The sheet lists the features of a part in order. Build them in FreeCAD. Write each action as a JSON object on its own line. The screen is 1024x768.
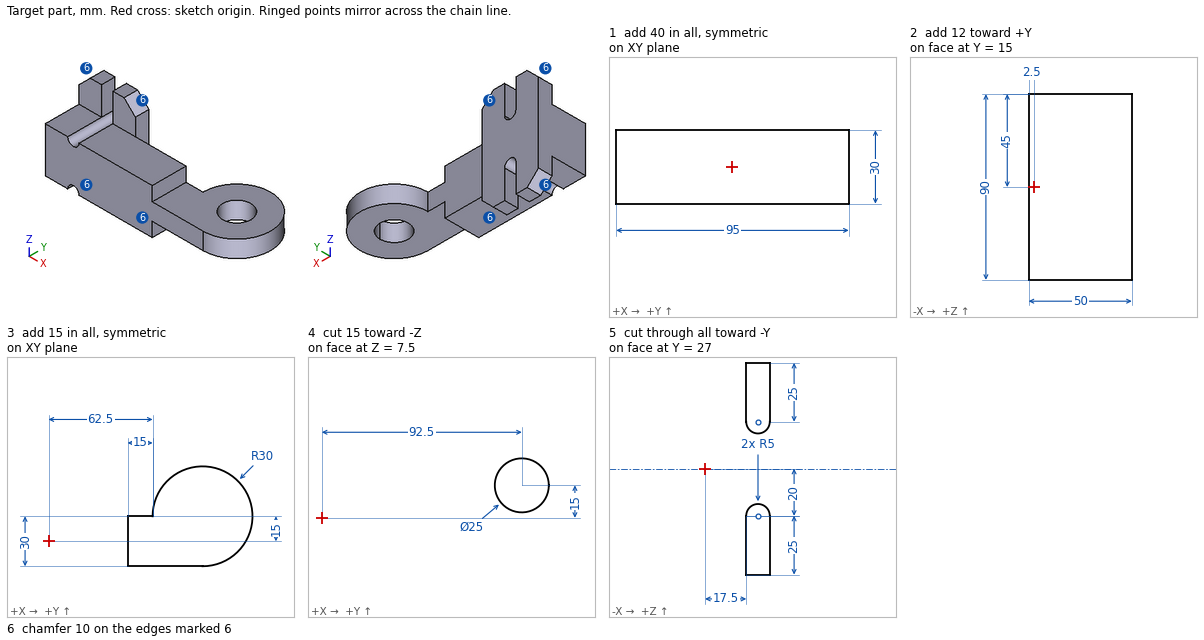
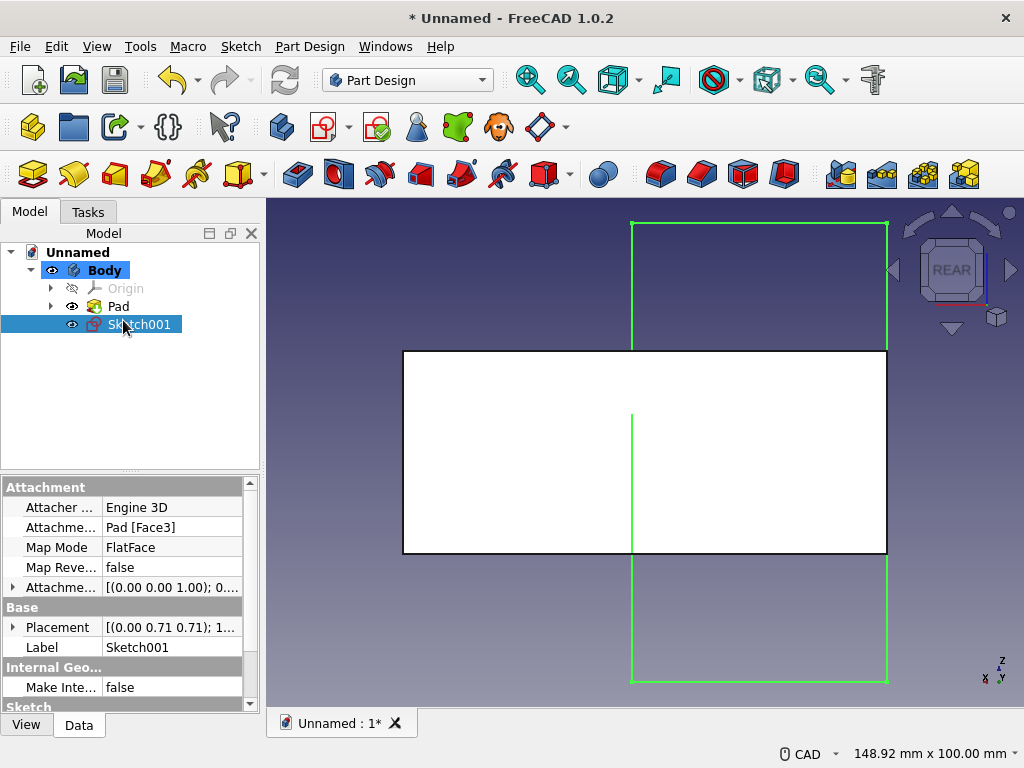
{"action": "left_click", "coordinate": [33, 174]}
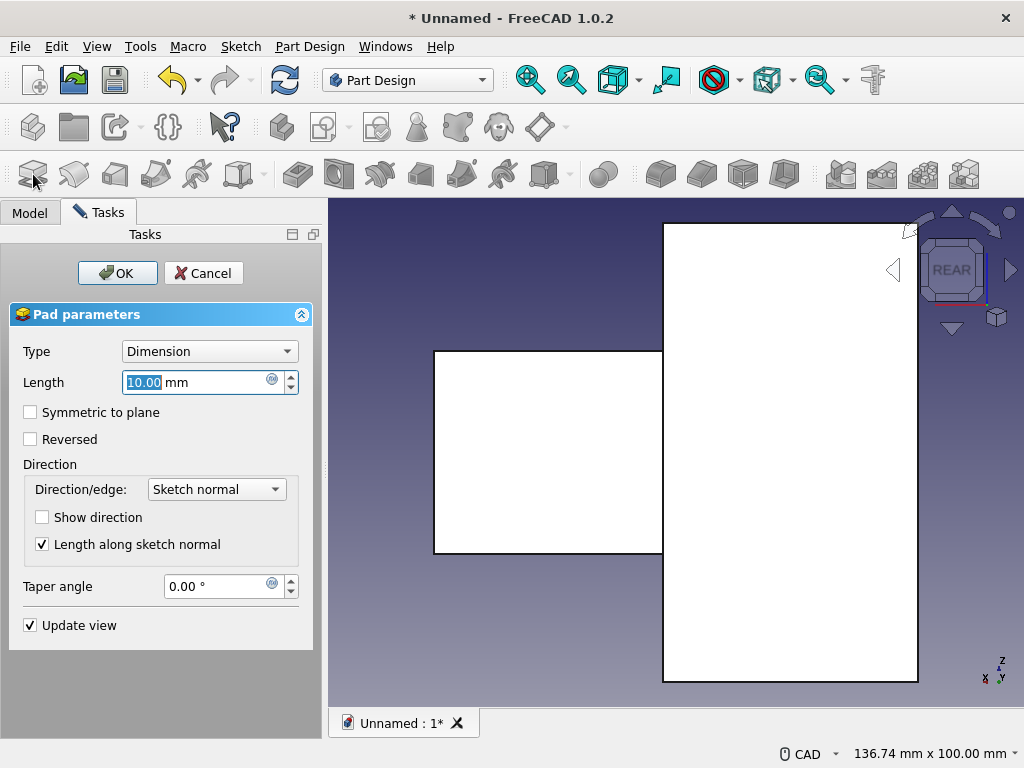
{"action": "type", "text": "12"}
{"action": "key", "text": "Tab"}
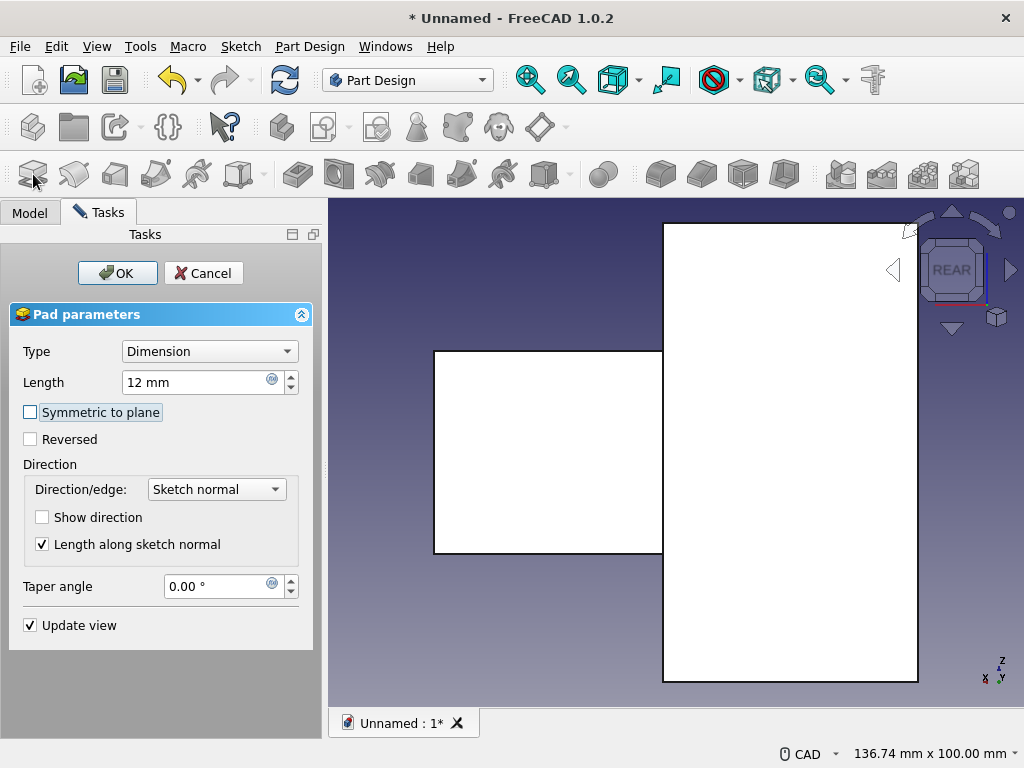
{"action": "left_click", "coordinate": [118, 273]}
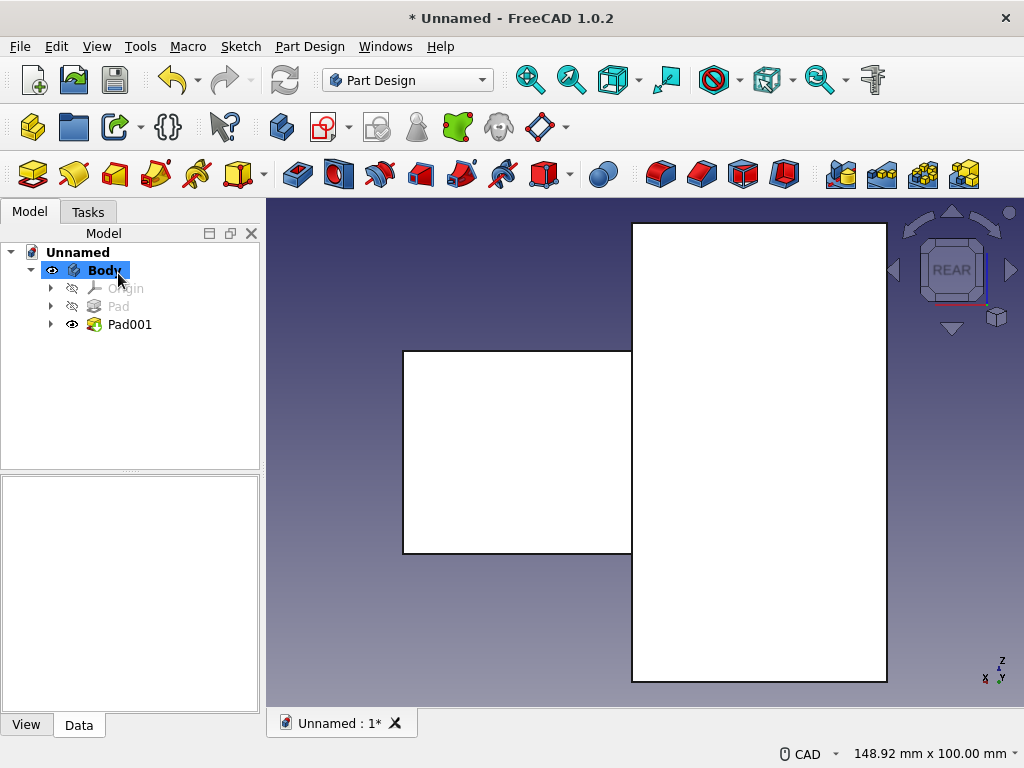
{"action": "left_click", "coordinate": [322, 128]}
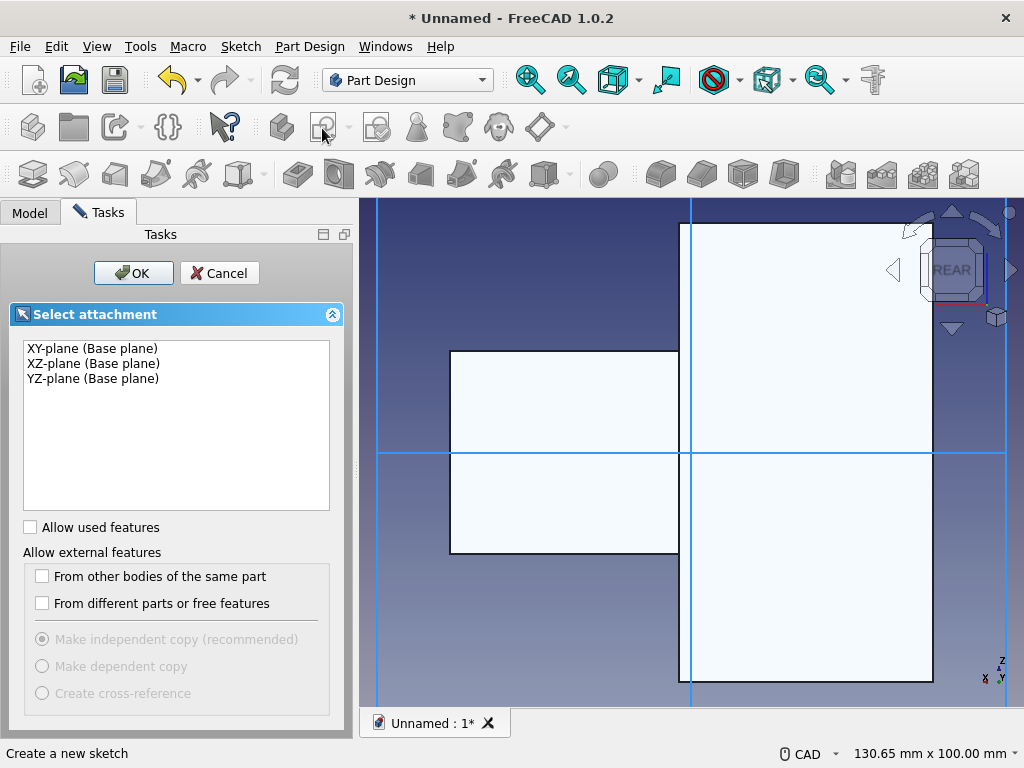
{"action": "left_click", "coordinate": [84, 348]}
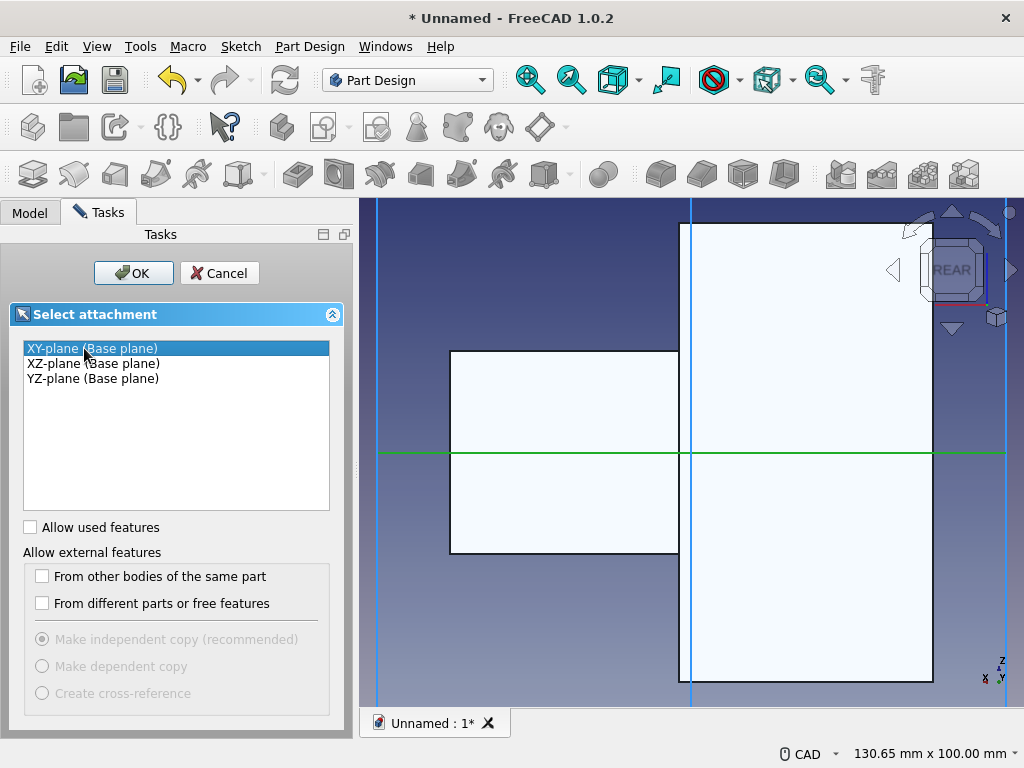
{"action": "left_click", "coordinate": [134, 273]}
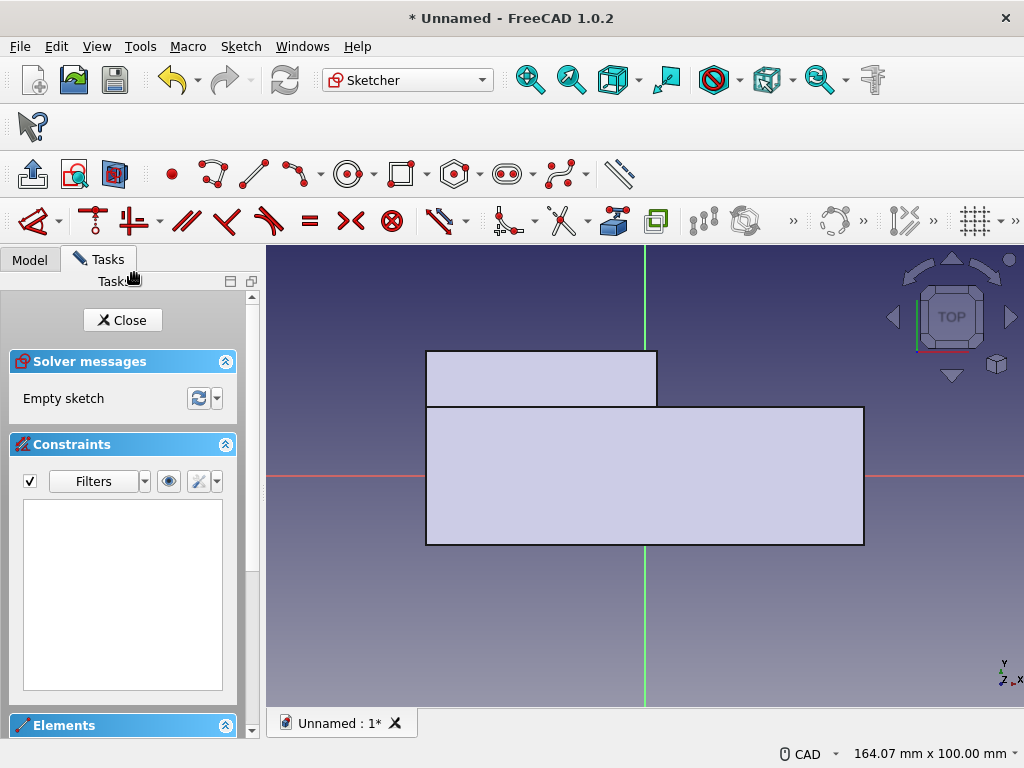
{"action": "left_click", "coordinate": [115, 174]}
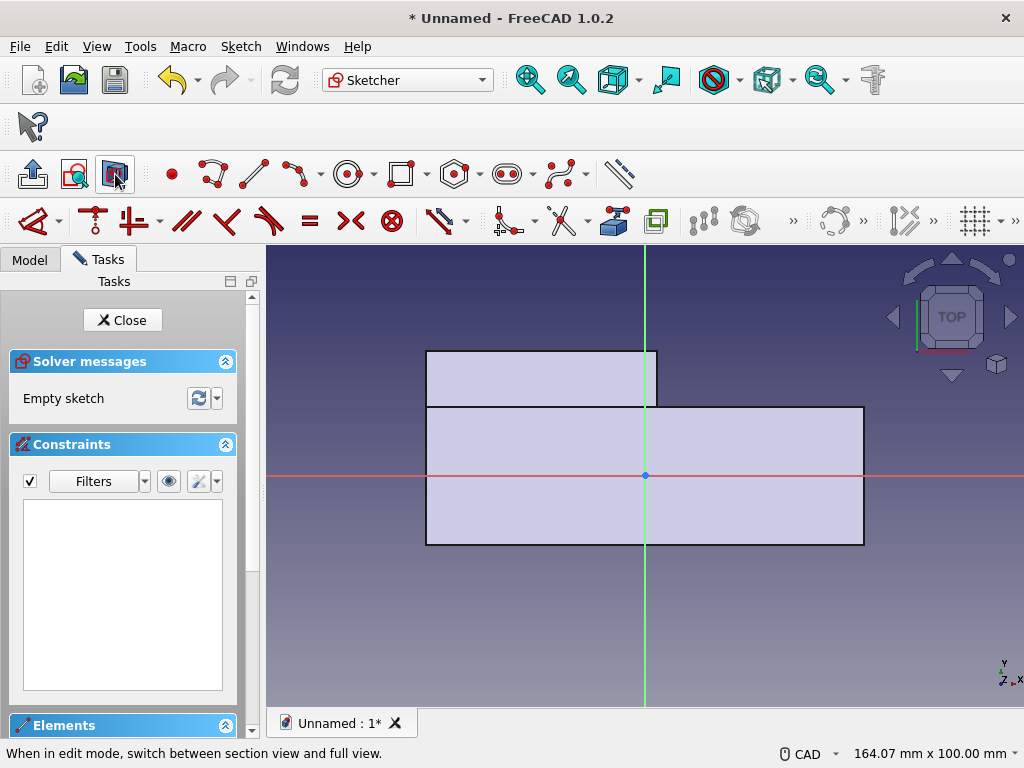
{"action": "scroll", "coordinate": [294, 536], "scroll_direction": "down", "scroll_amount": 3}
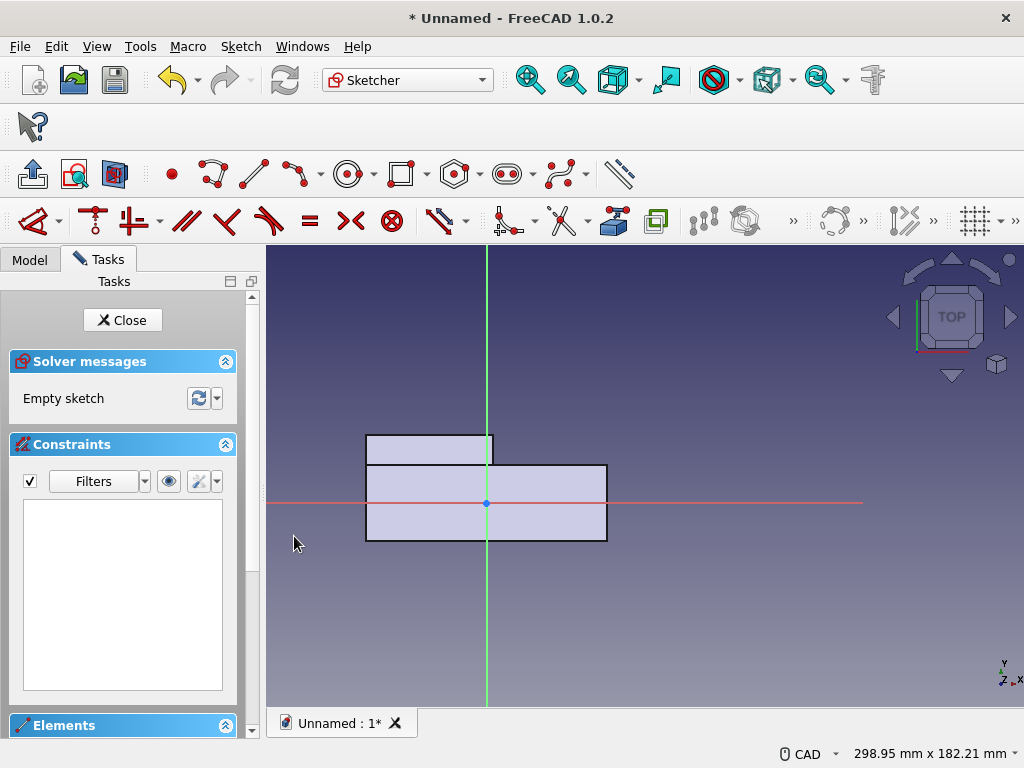
{"action": "scroll", "coordinate": [741, 477], "scroll_direction": "up", "scroll_amount": 2}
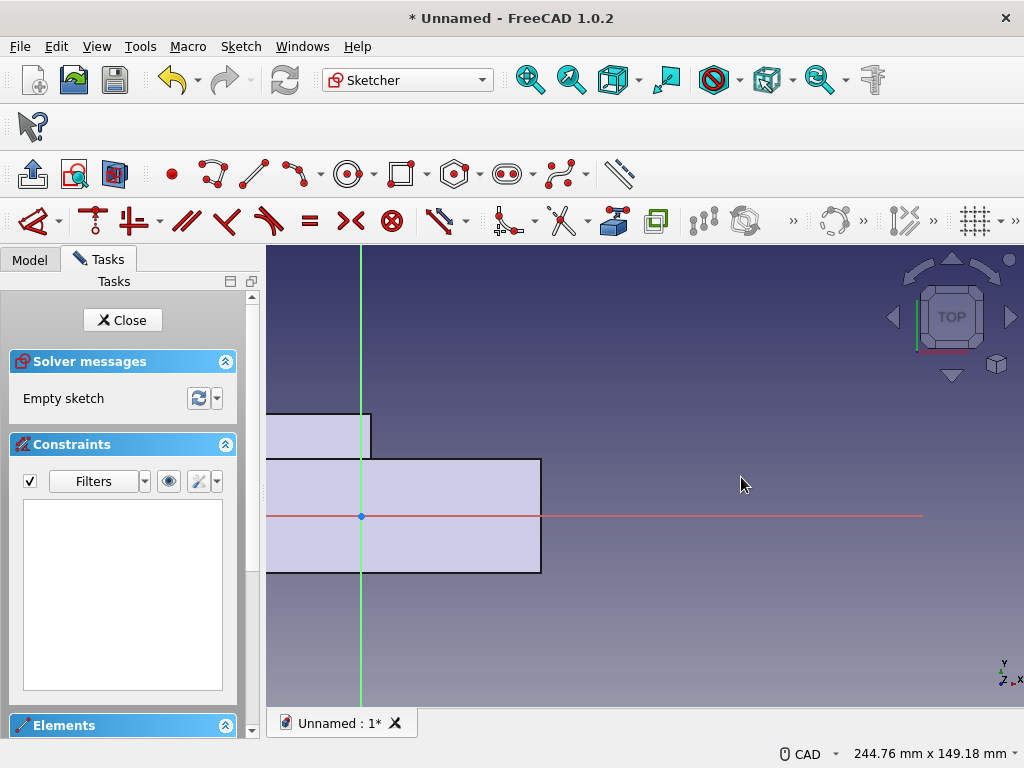
{"action": "key", "text": "g m"}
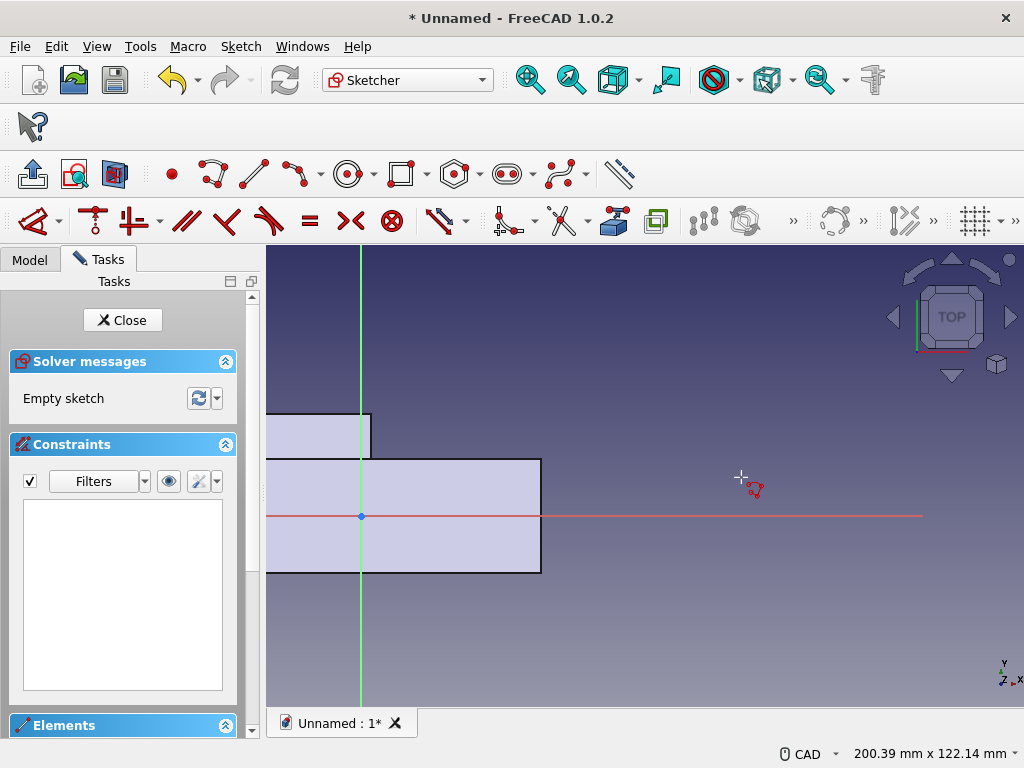
{"action": "left_click", "coordinate": [598, 459]}
{"action": "left_click", "coordinate": [541, 459]}
{"action": "left_click", "coordinate": [541, 573]}
{"action": "left_click", "coordinate": [711, 573]}
{"action": "right_click", "coordinate": [711, 573]}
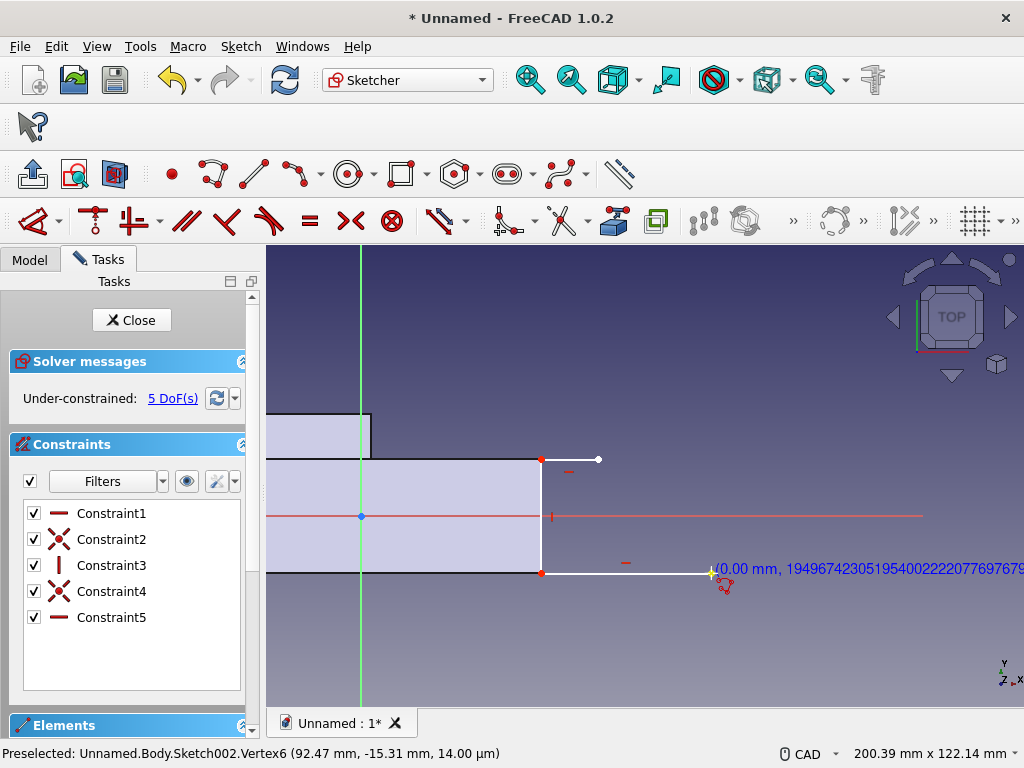
{"action": "left_click", "coordinate": [294, 174]}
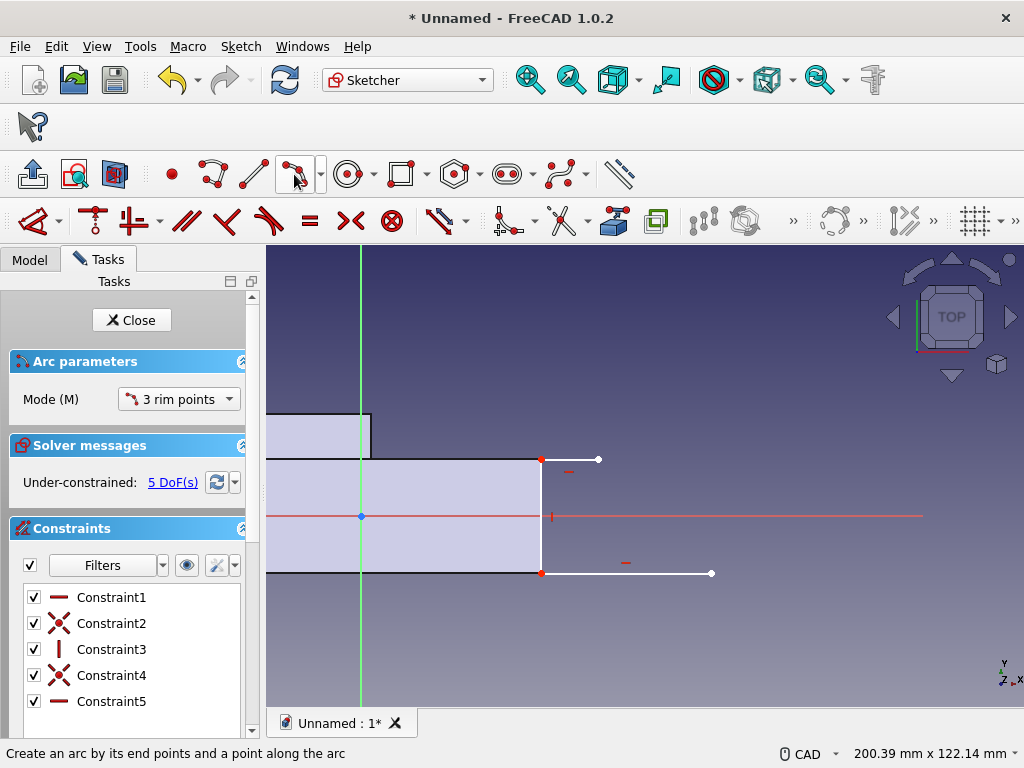
{"action": "left_click", "coordinate": [711, 574]}
{"action": "left_click", "coordinate": [598, 460]}
{"action": "left_click", "coordinate": [791, 379]}
{"action": "key", "text": "Escape"}